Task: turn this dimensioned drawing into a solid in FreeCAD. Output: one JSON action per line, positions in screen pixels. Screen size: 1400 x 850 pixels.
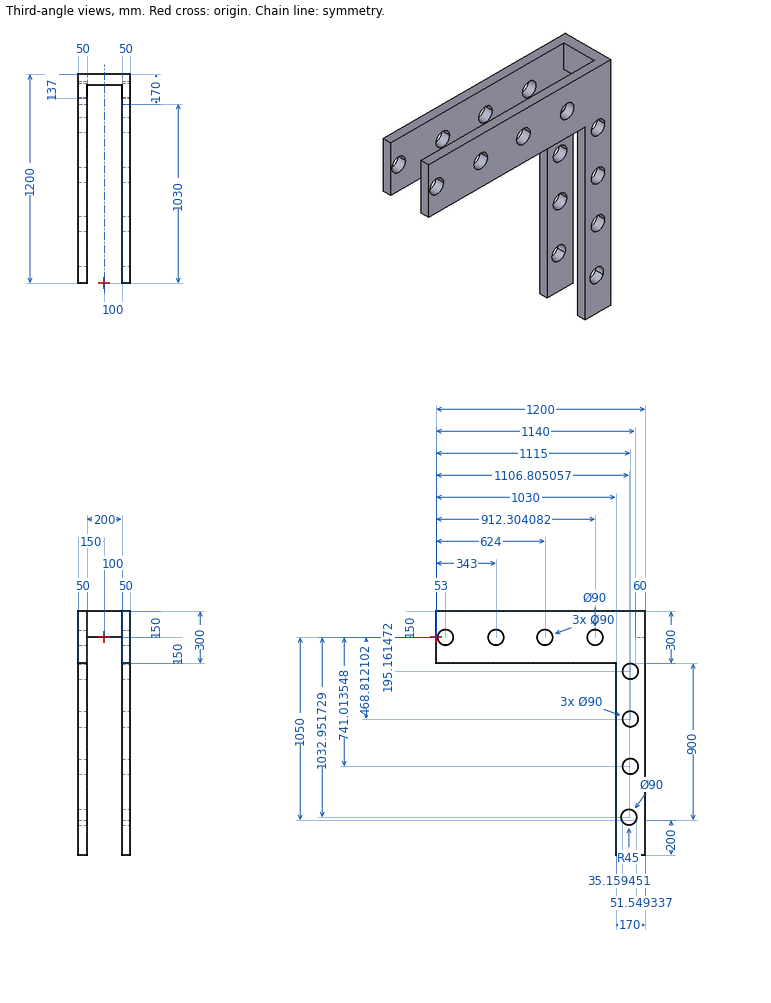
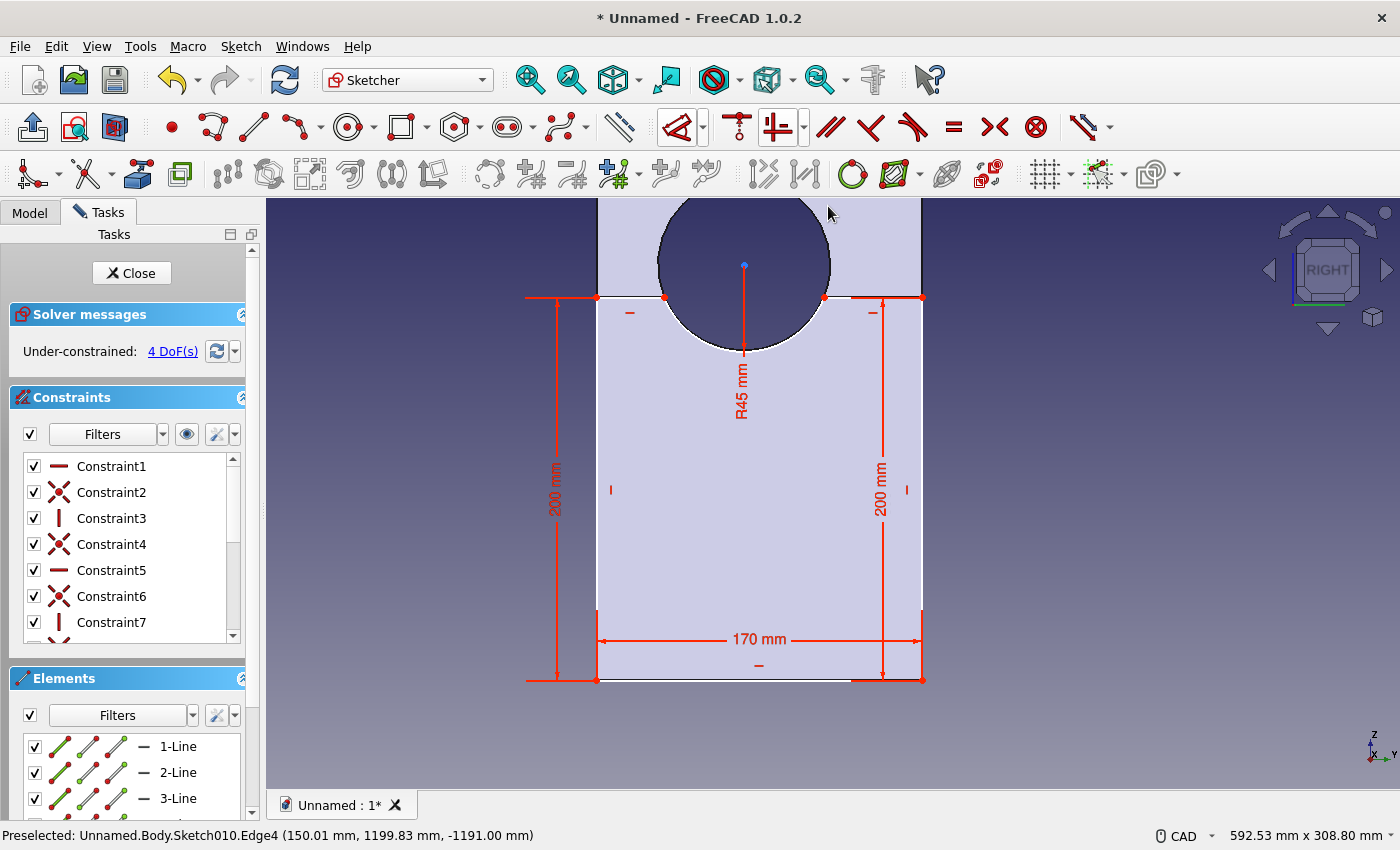
{"action": "left_click", "coordinate": [664, 298]}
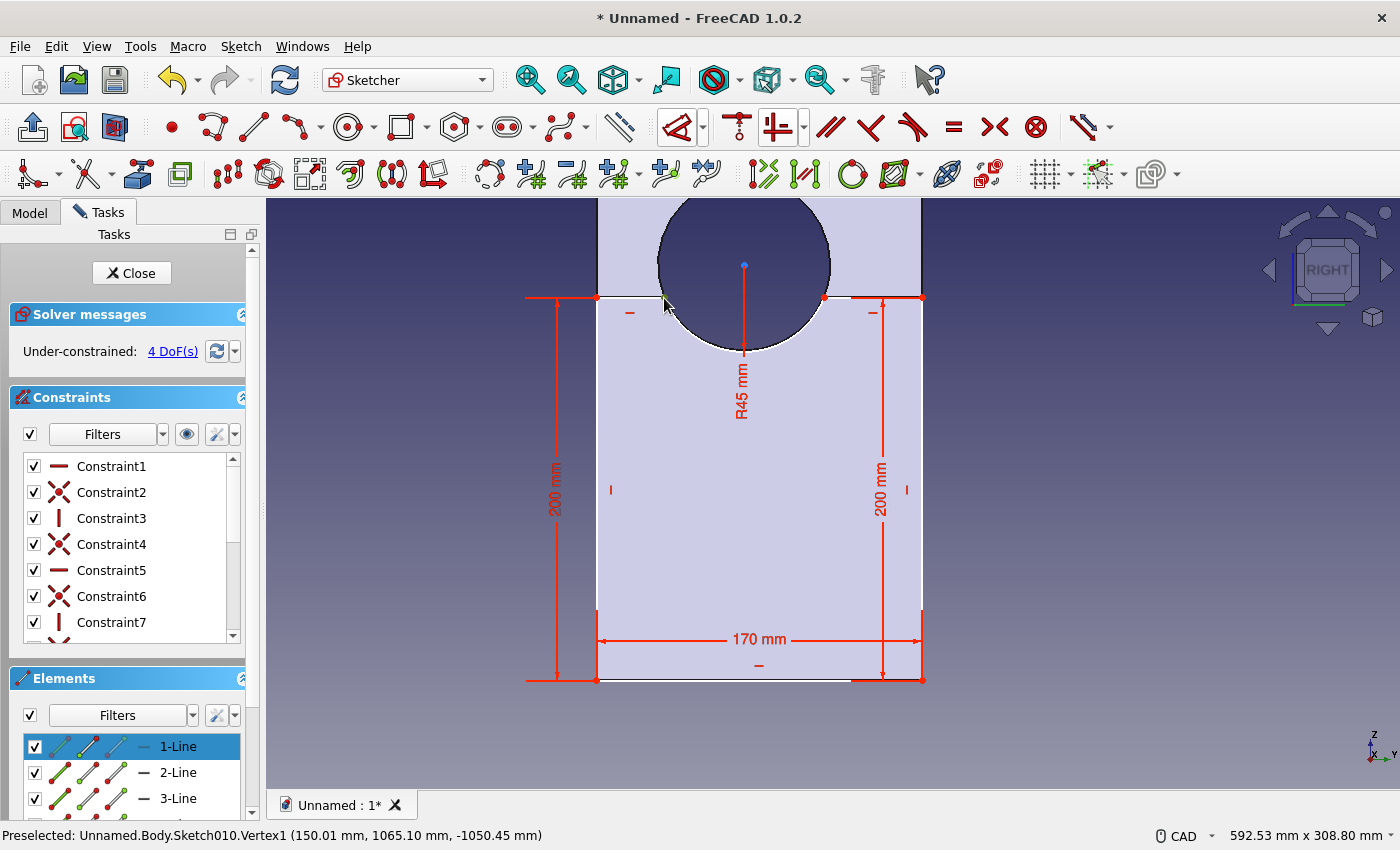
{"action": "left_click", "coordinate": [702, 128]}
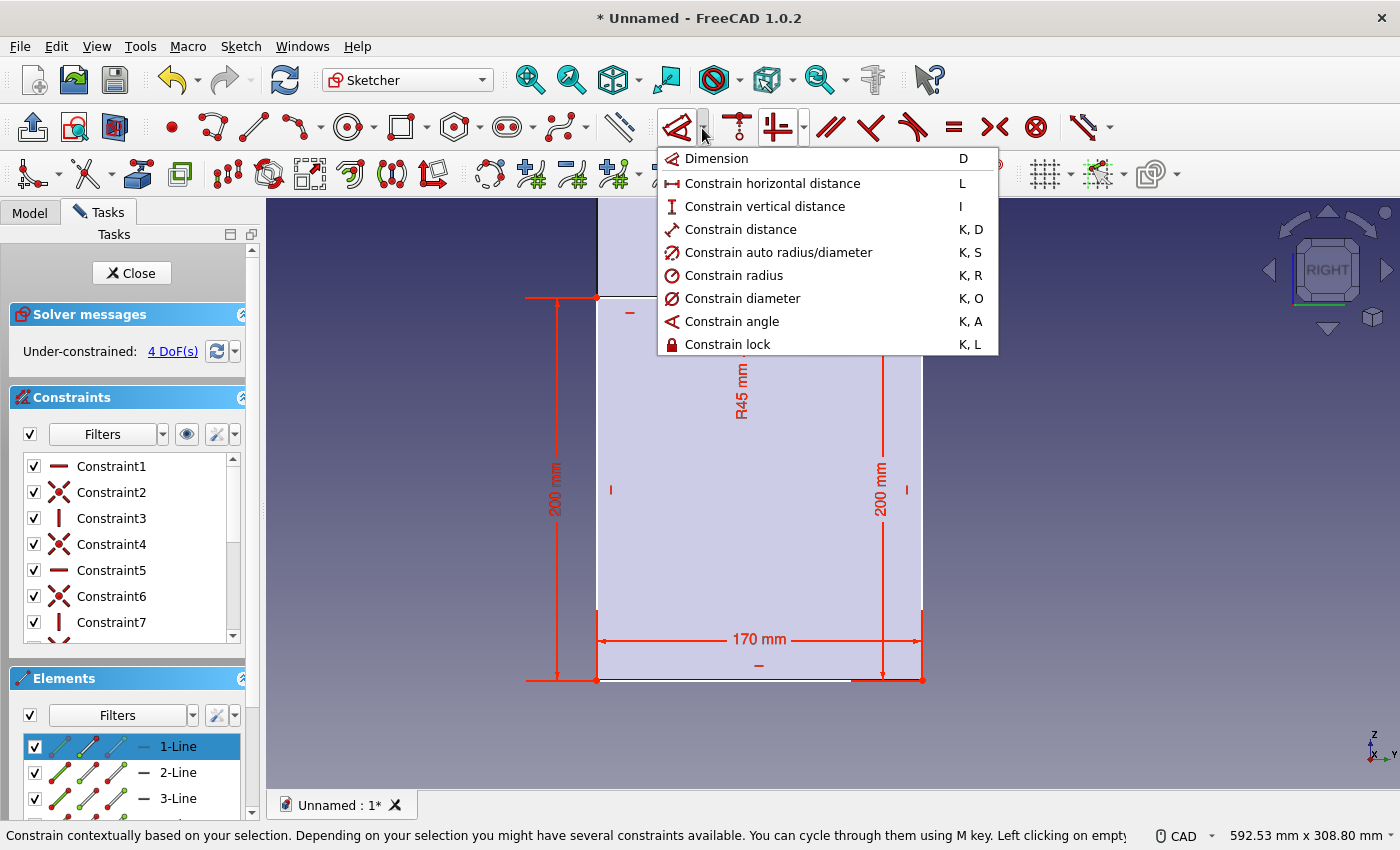
{"action": "left_click", "coordinate": [828, 206]}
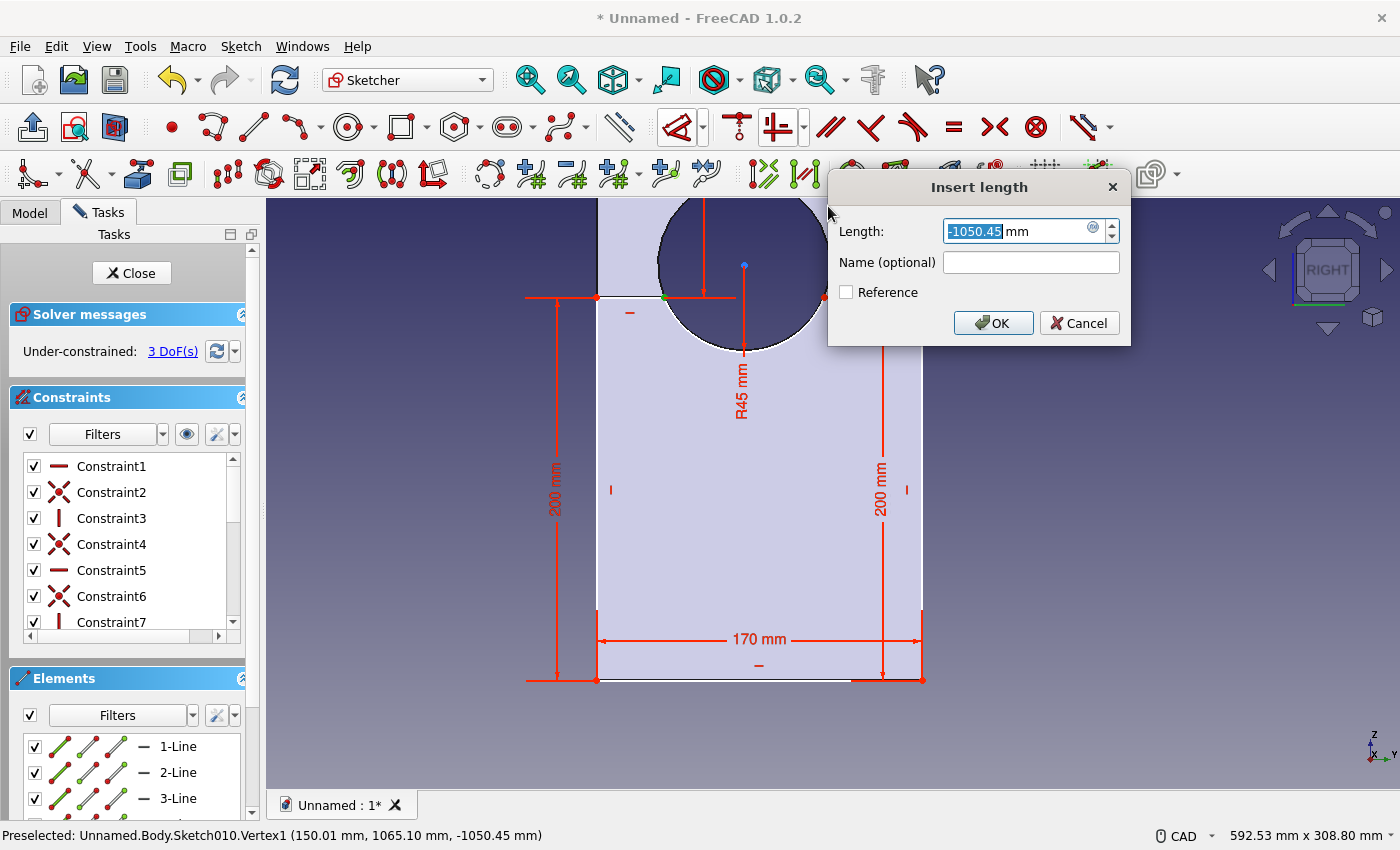
{"action": "type", "text": "-1050"}
{"action": "key", "text": "Return"}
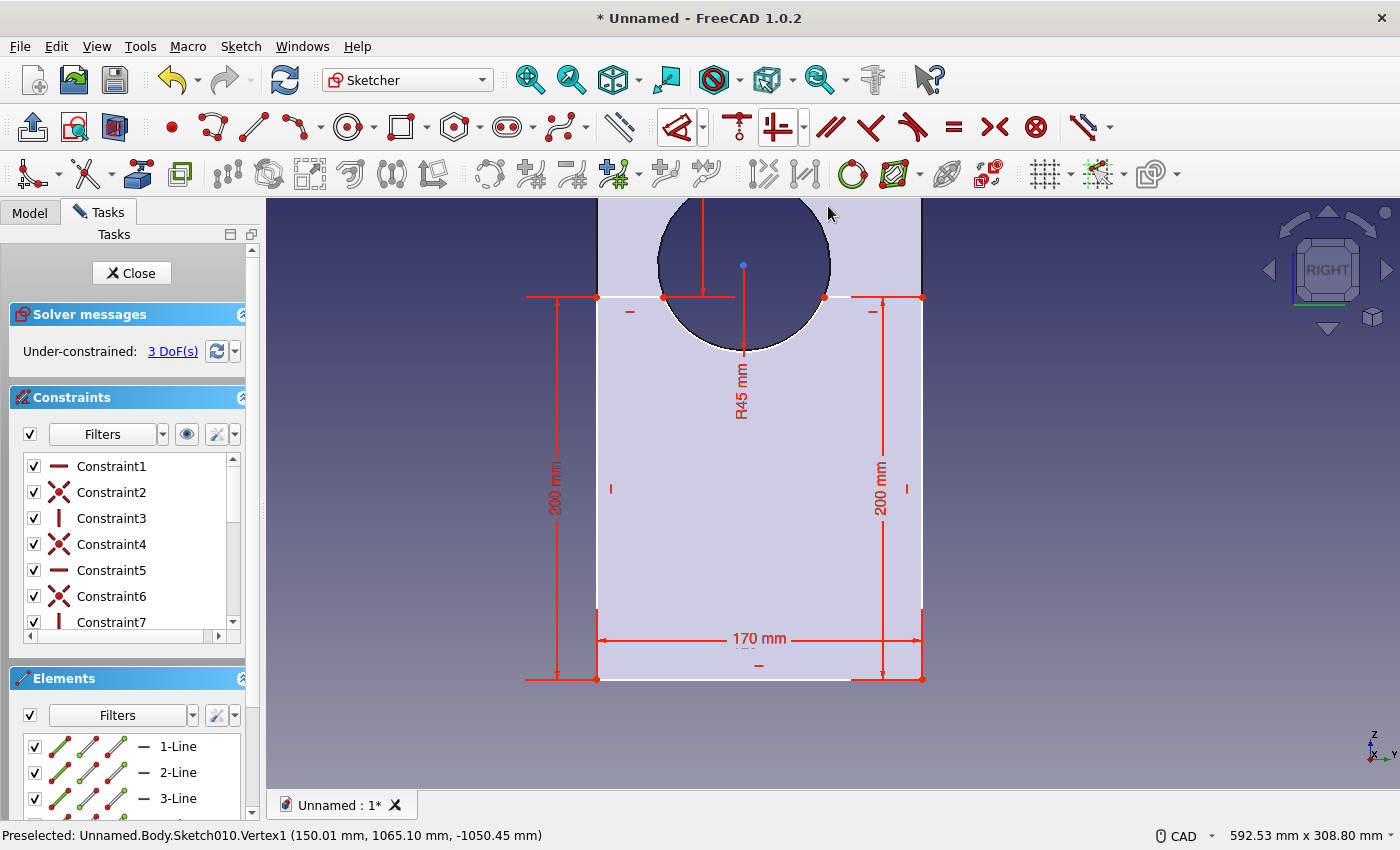
{"action": "left_click", "coordinate": [597, 297]}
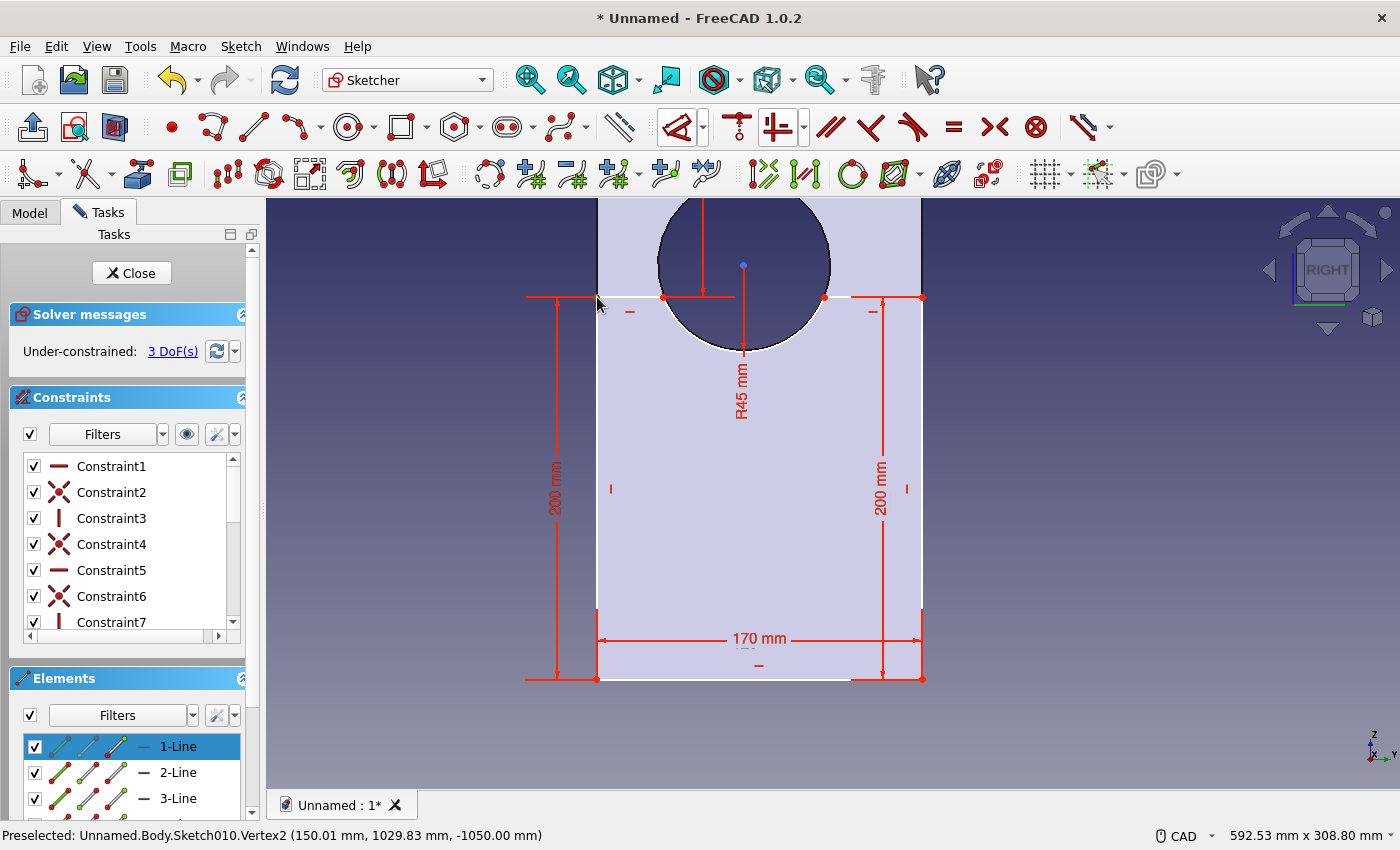
{"action": "key", "text": "l"}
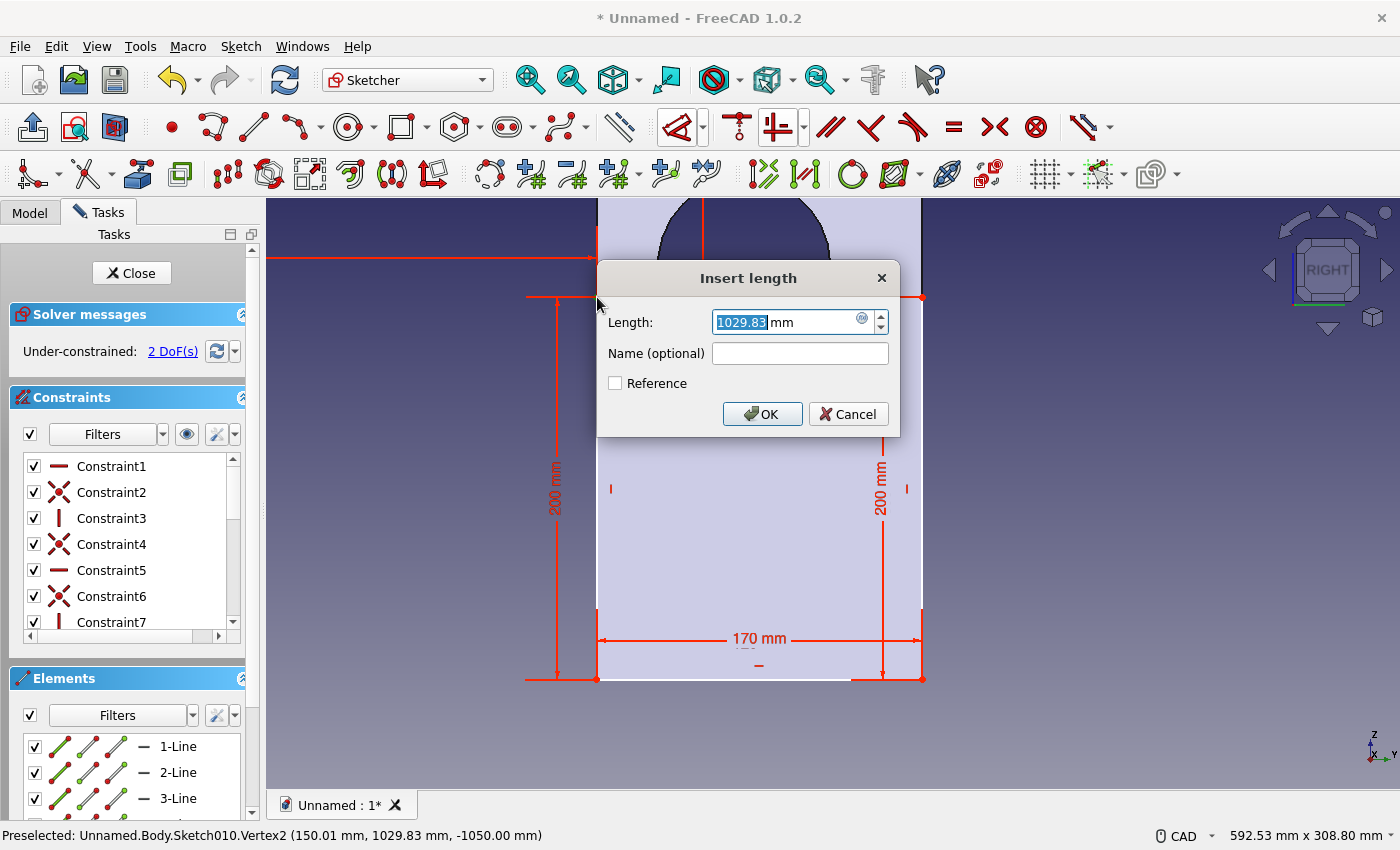
{"action": "type", "text": "1030"}
{"action": "key", "text": "Return"}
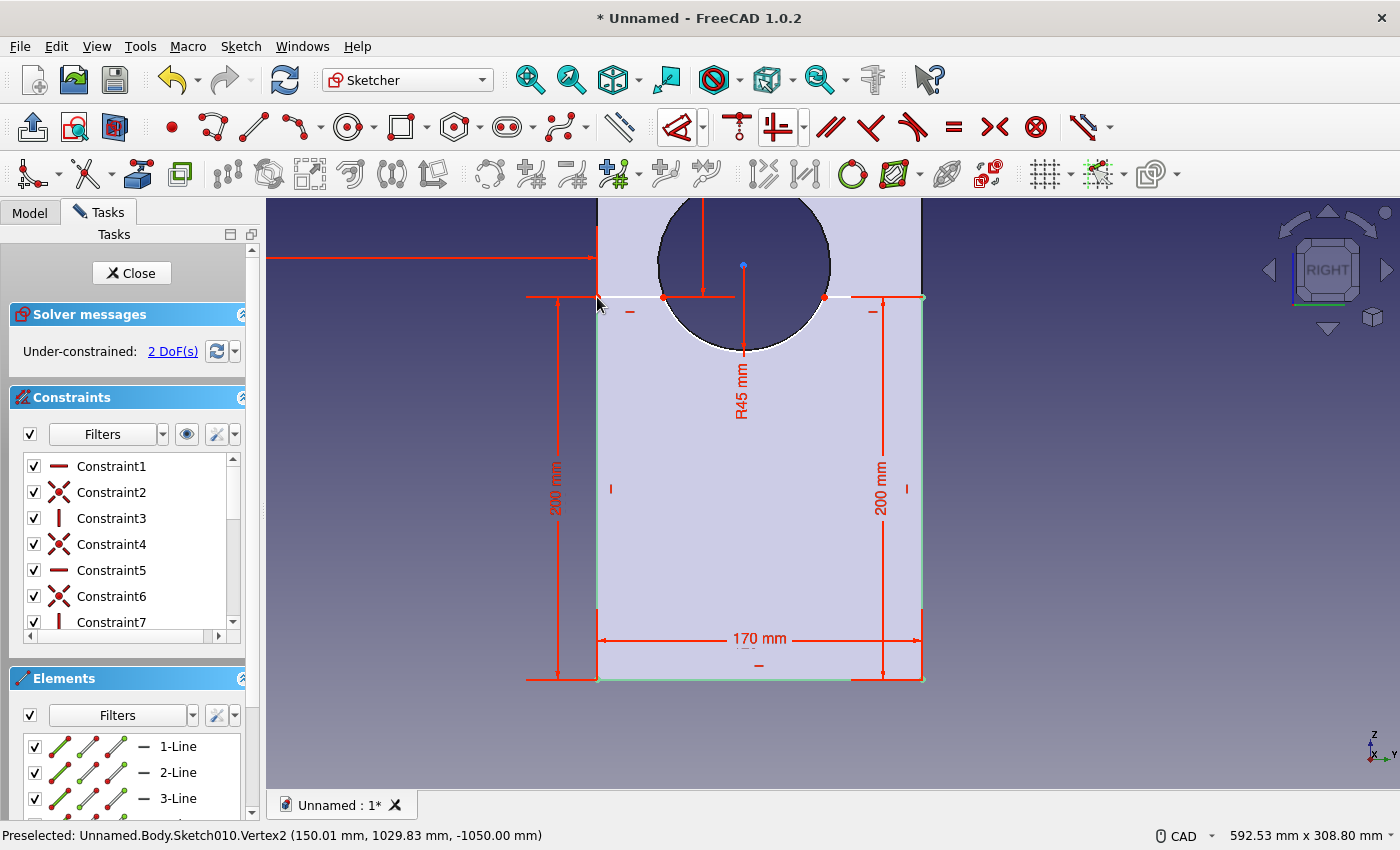
{"action": "left_click", "coordinate": [644, 297]}